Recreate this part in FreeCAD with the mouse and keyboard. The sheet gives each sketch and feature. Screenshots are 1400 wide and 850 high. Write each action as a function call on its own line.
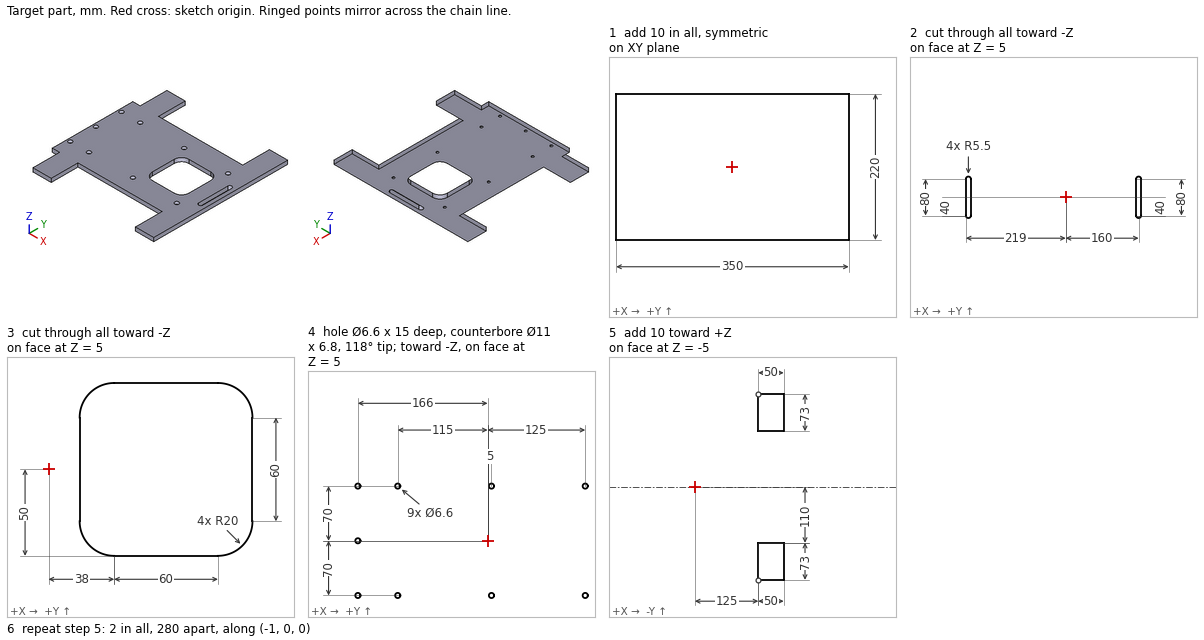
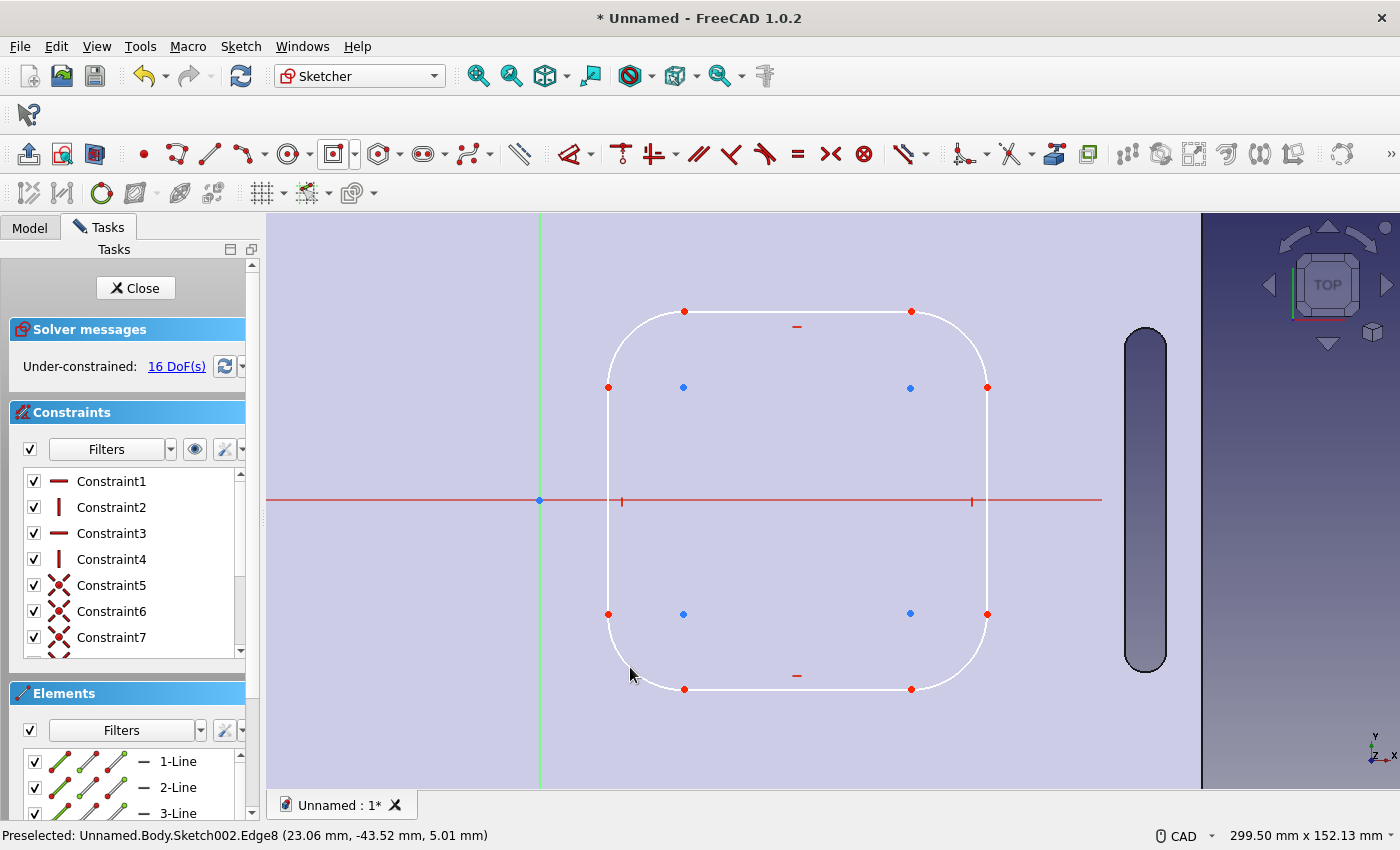
click(752, 690)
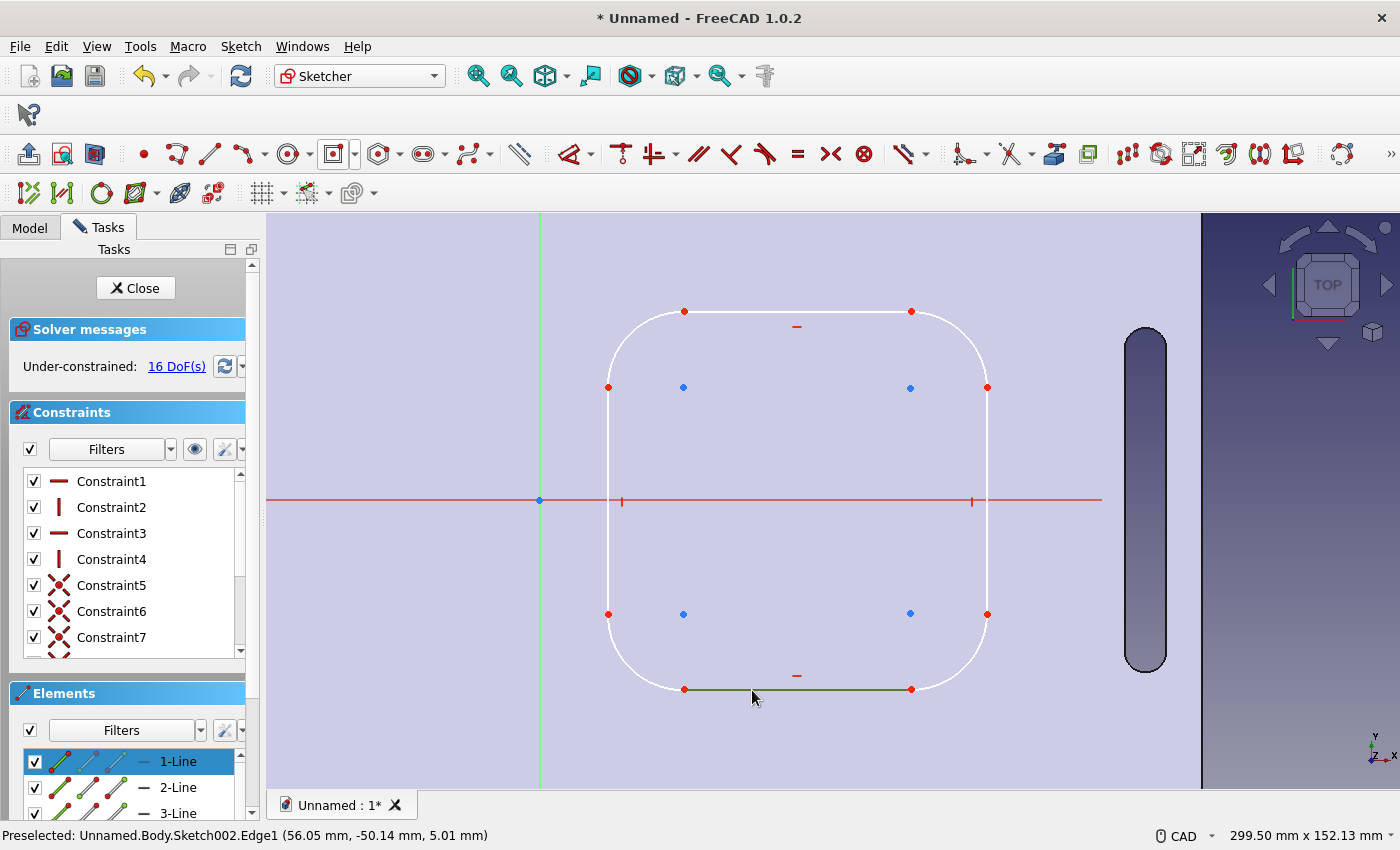
click(945, 682)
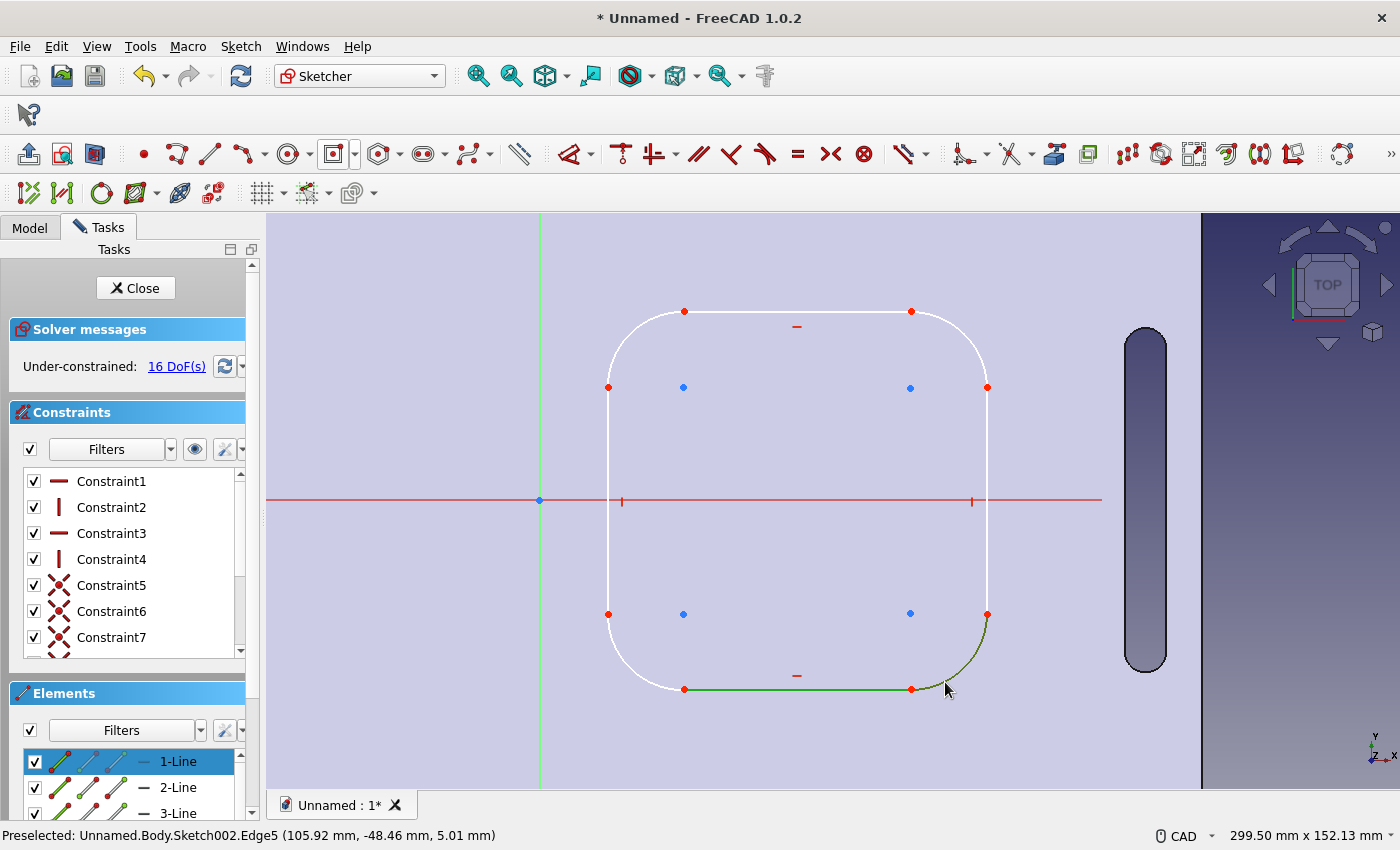
key(t)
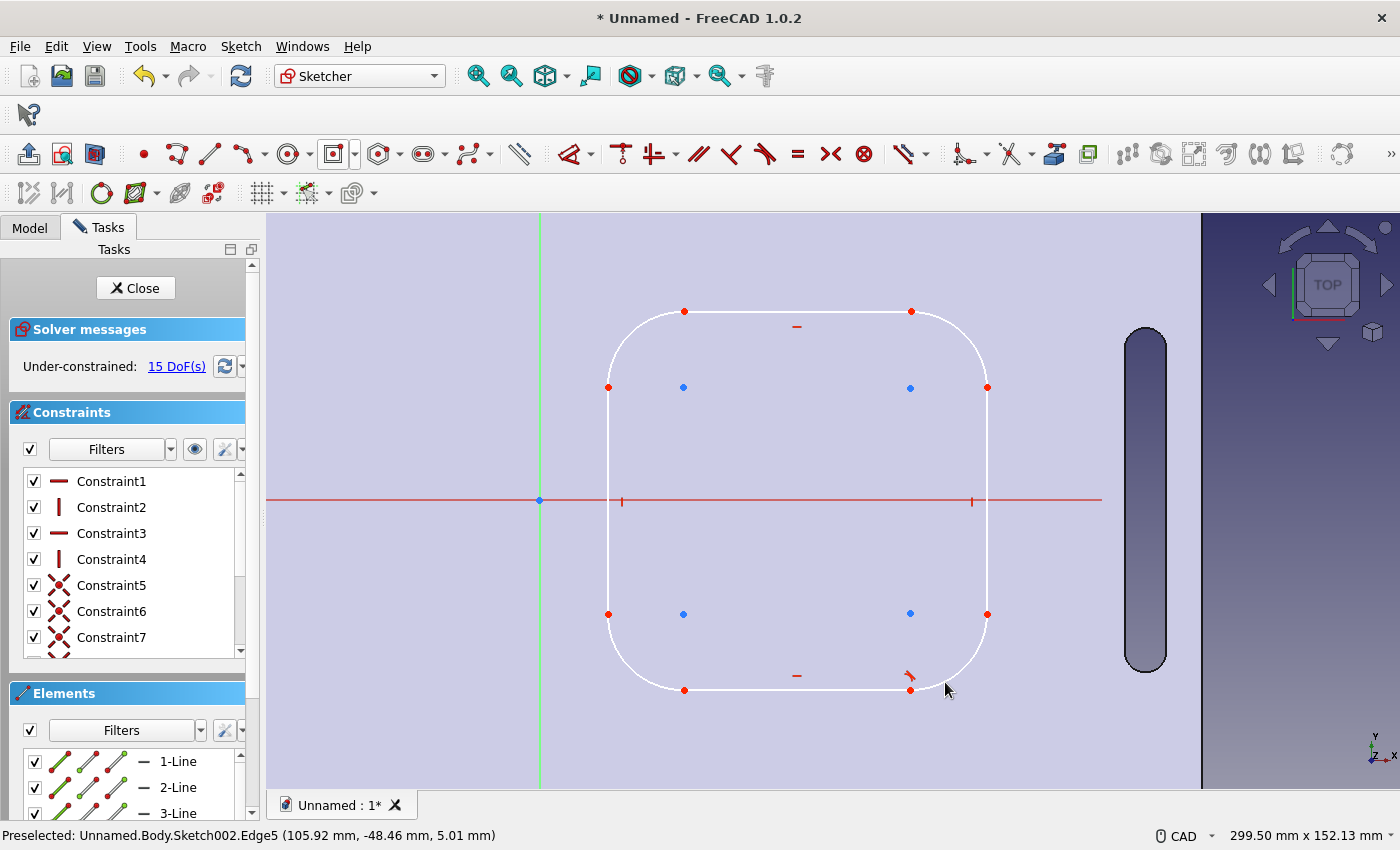
click(752, 690)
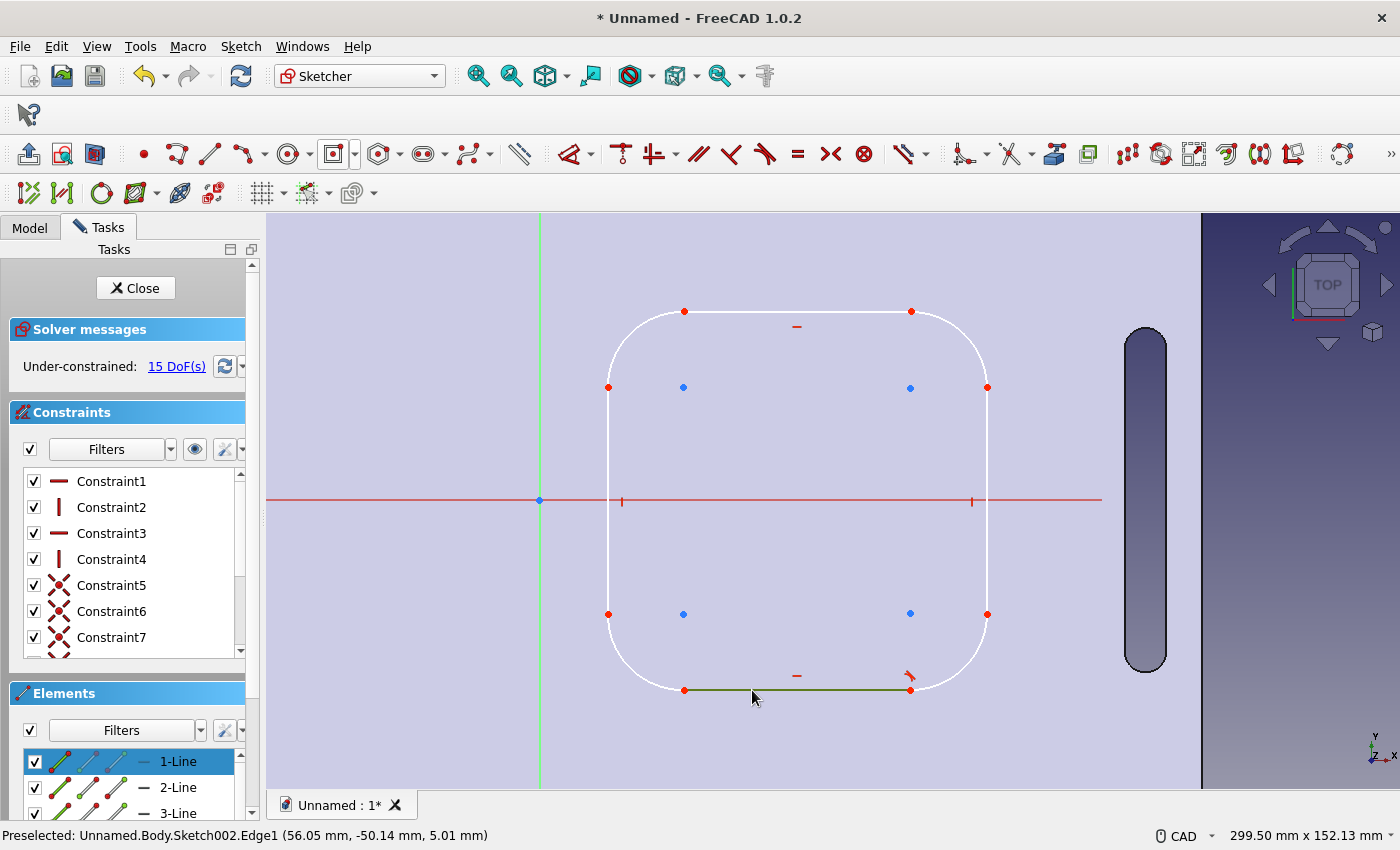
click(616, 649)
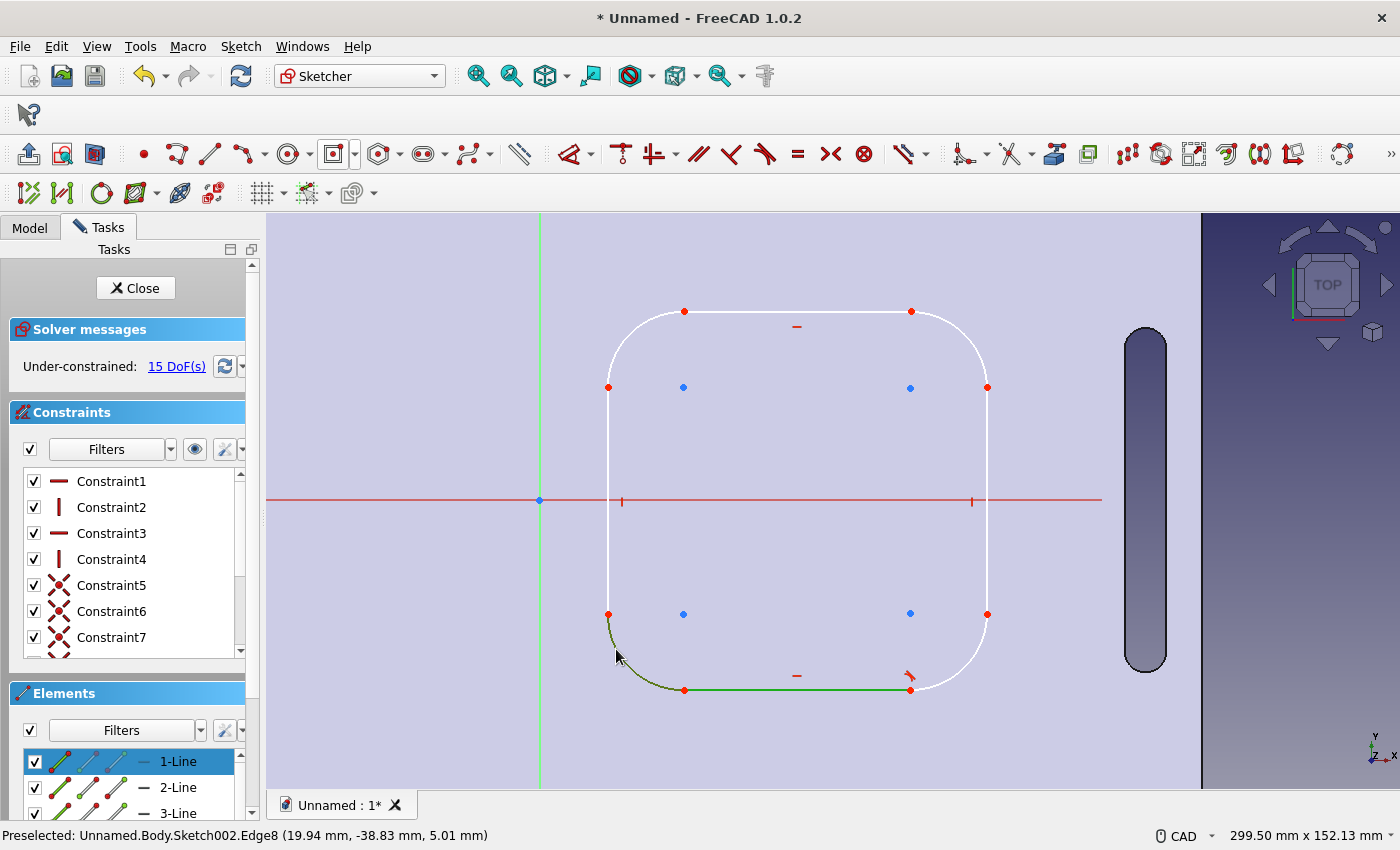
click(765, 154)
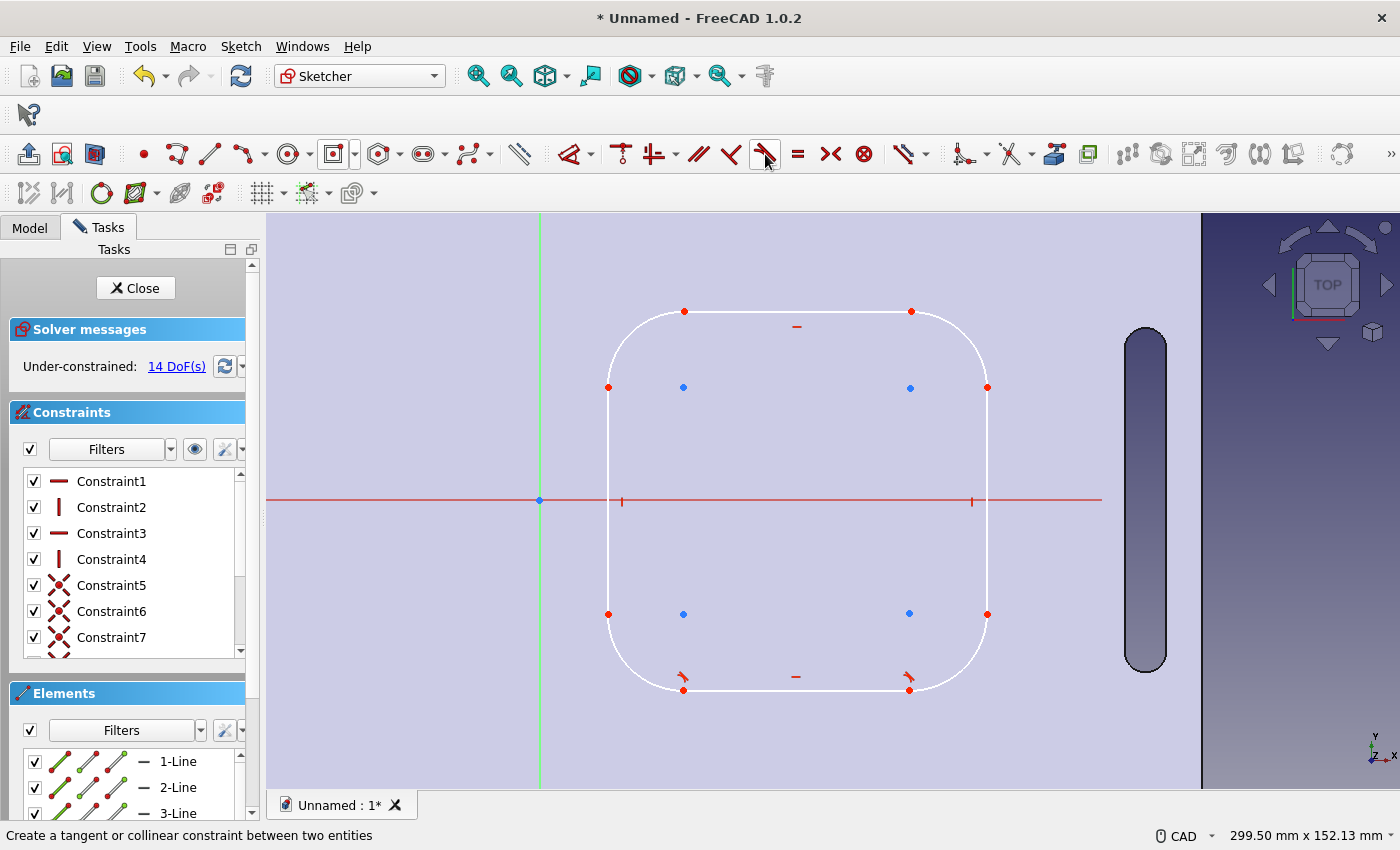
click(987, 547)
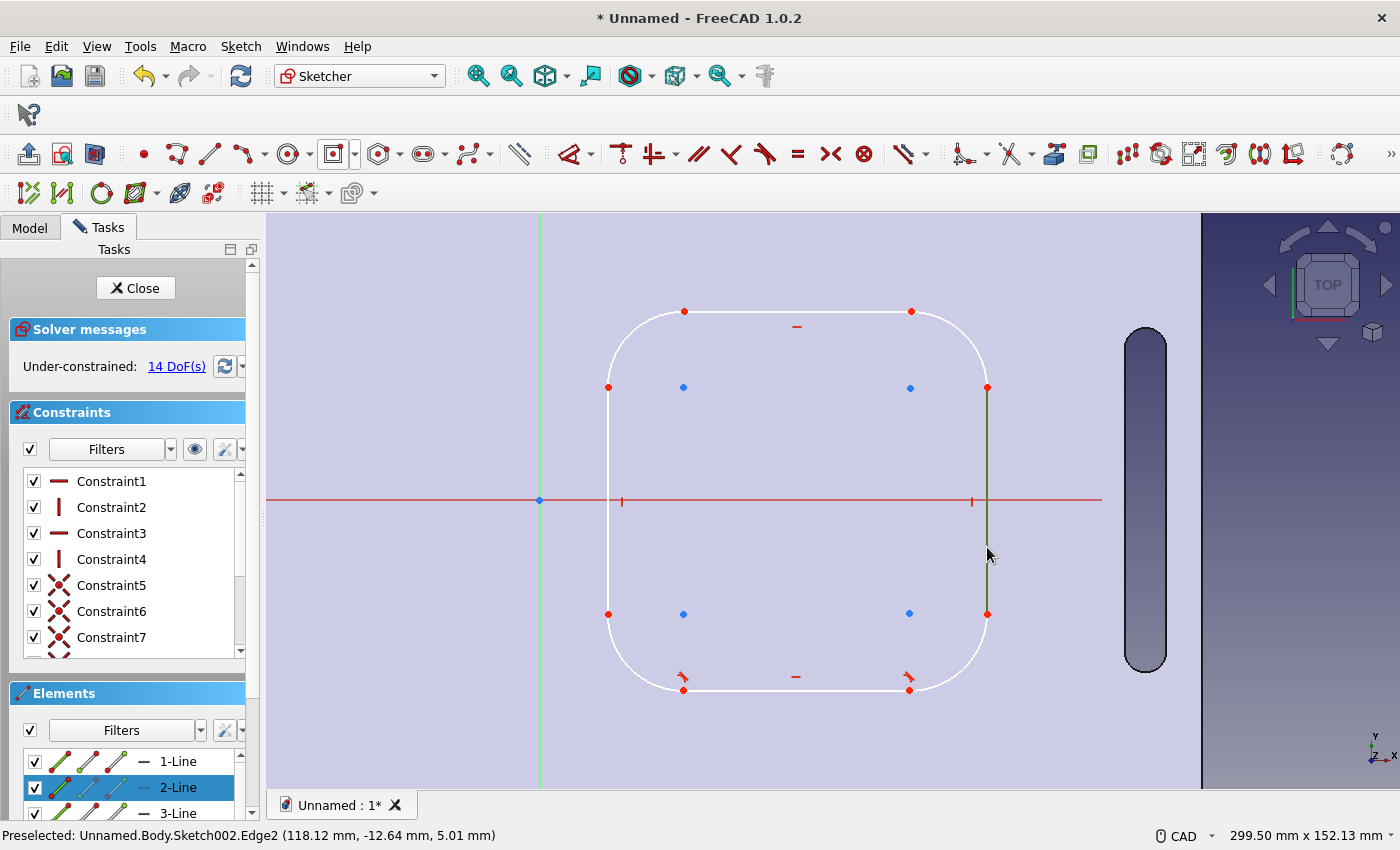
click(944, 683)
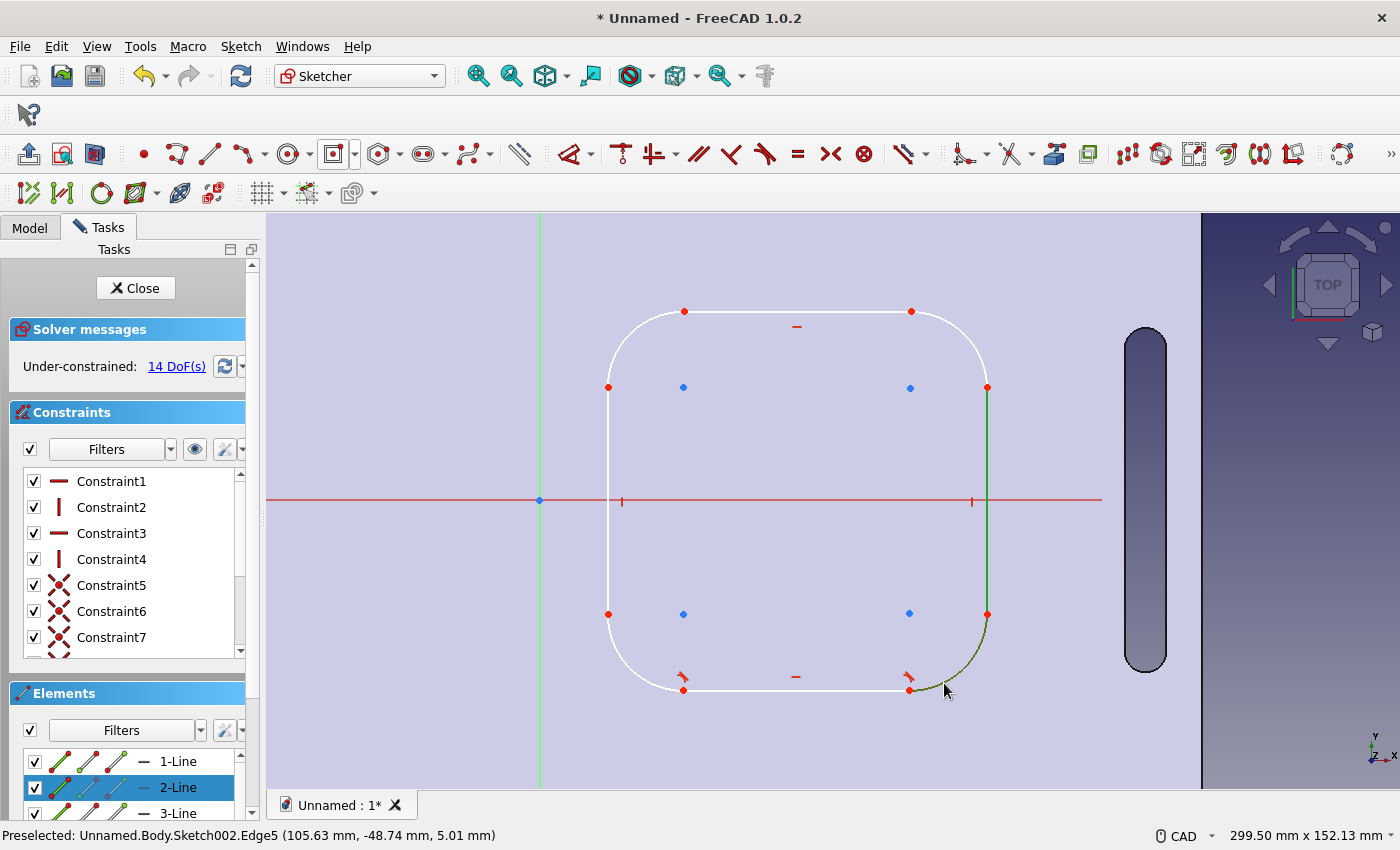
click(765, 154)